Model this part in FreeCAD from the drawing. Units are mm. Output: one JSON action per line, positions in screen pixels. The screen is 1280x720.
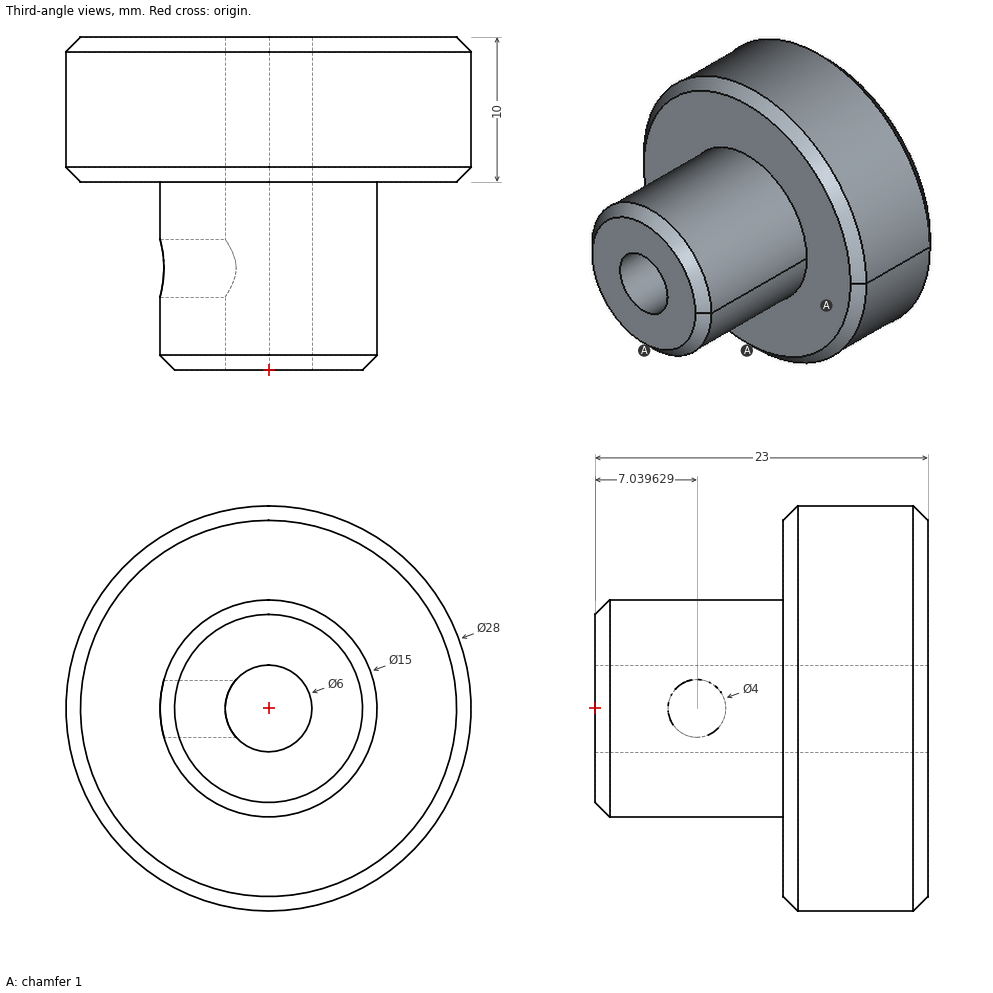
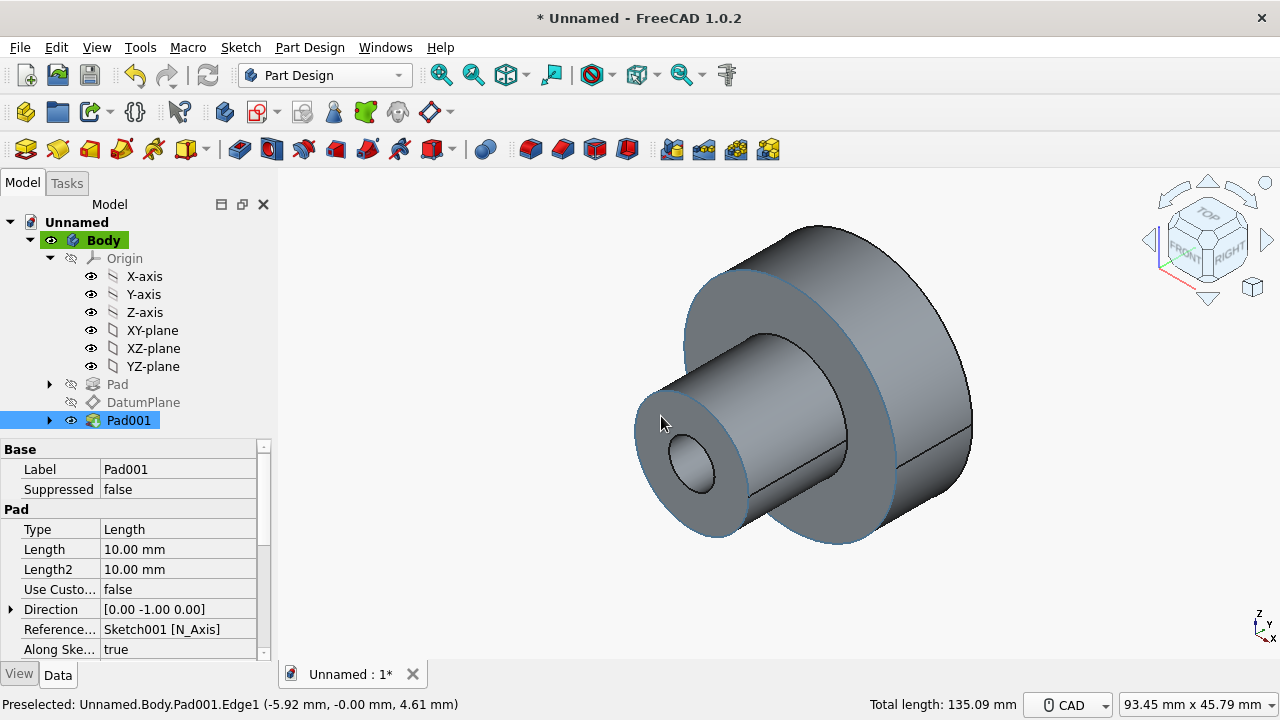
{"action": "key", "text": "2"}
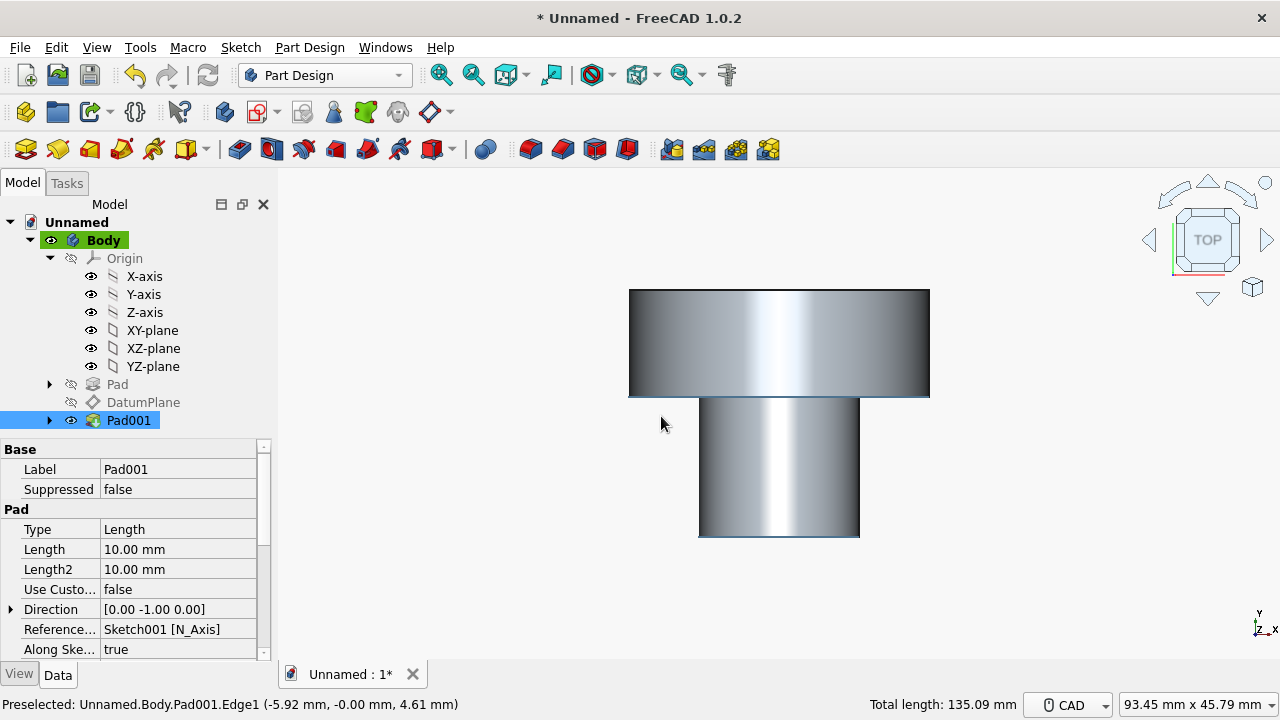
{"action": "left_click", "coordinate": [658, 289], "text": "ctrl"}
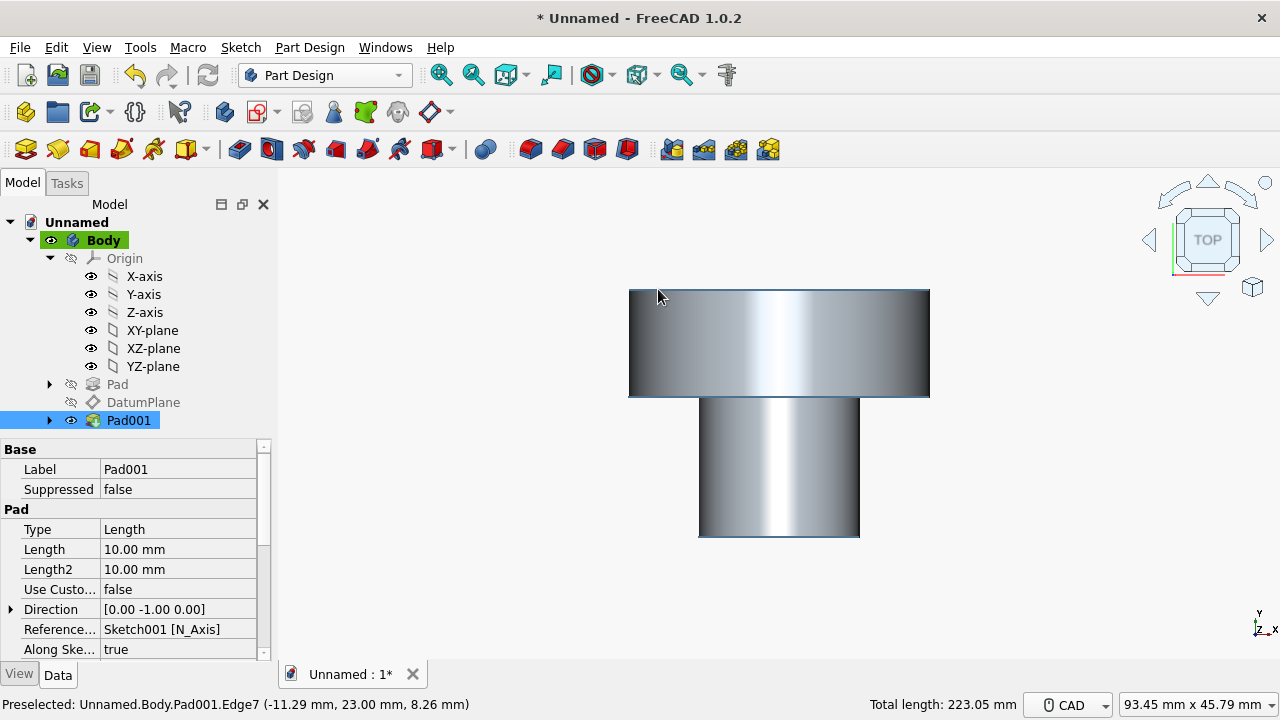
{"action": "left_click", "coordinate": [564, 150]}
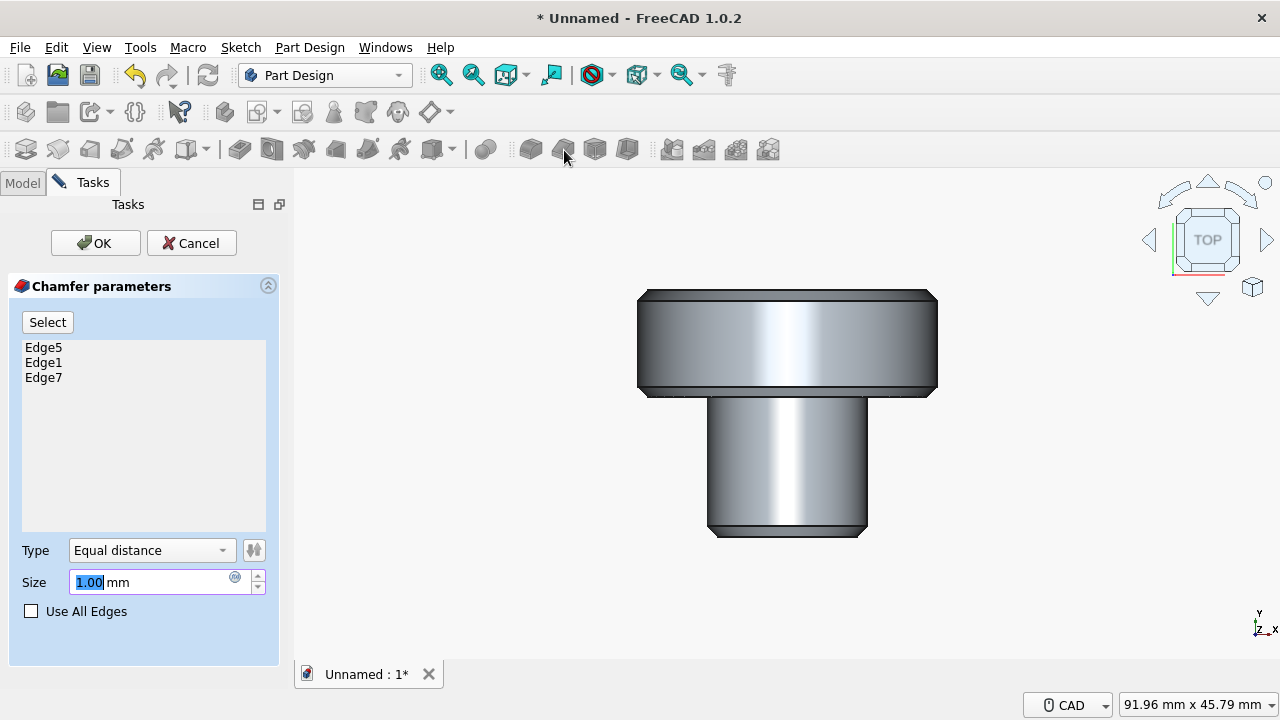
{"action": "type", "text": "1"}
{"action": "key", "text": "Tab"}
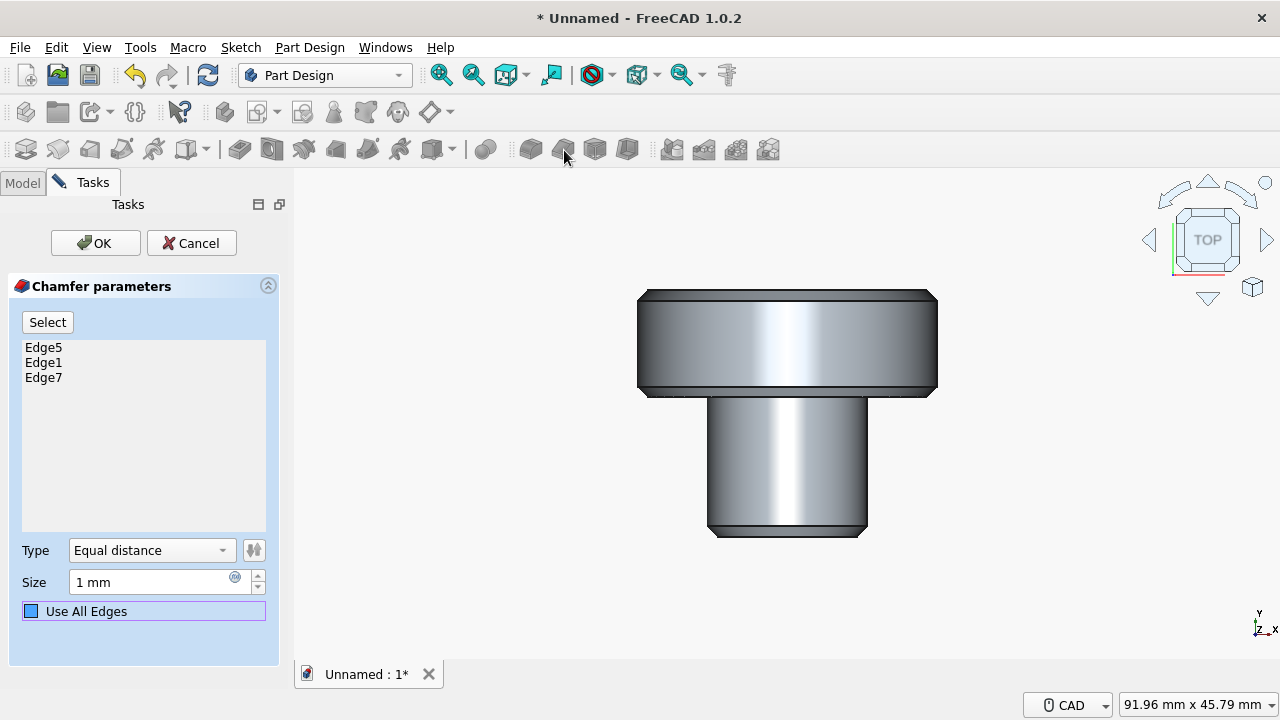
{"action": "left_click", "coordinate": [96, 243]}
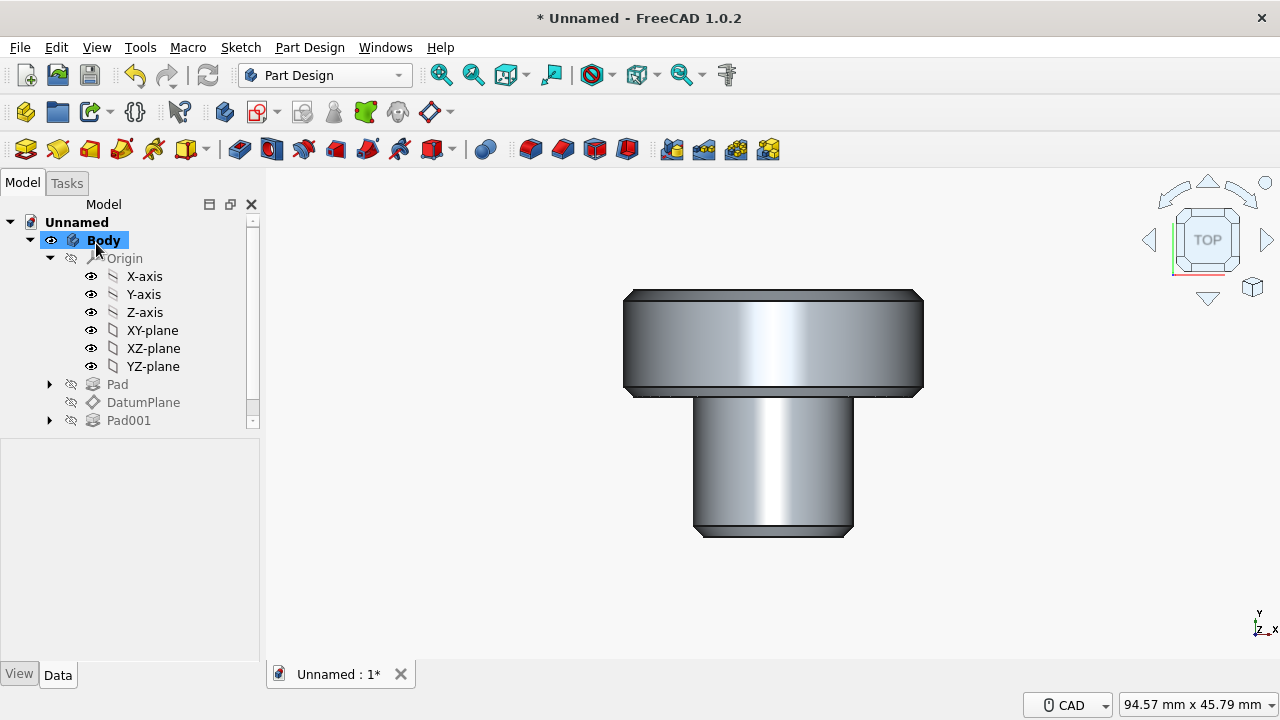
{"action": "left_click", "coordinate": [258, 112]}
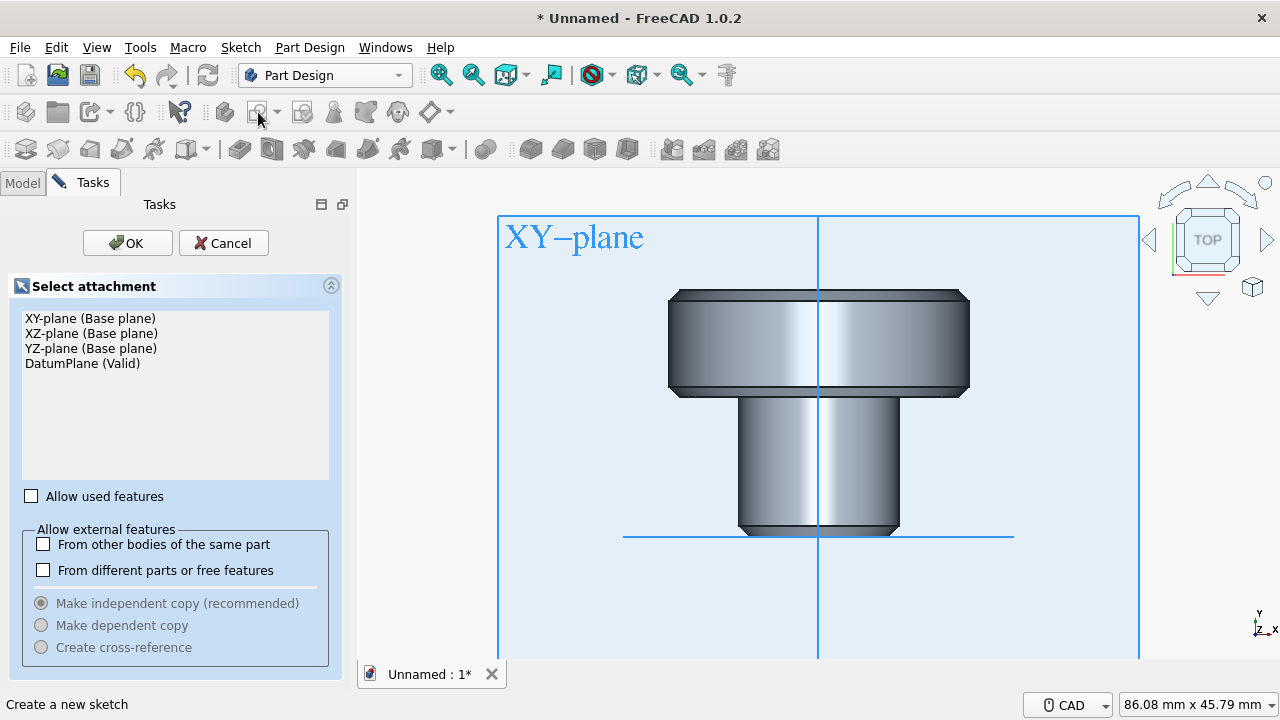
{"action": "left_click", "coordinate": [82, 348]}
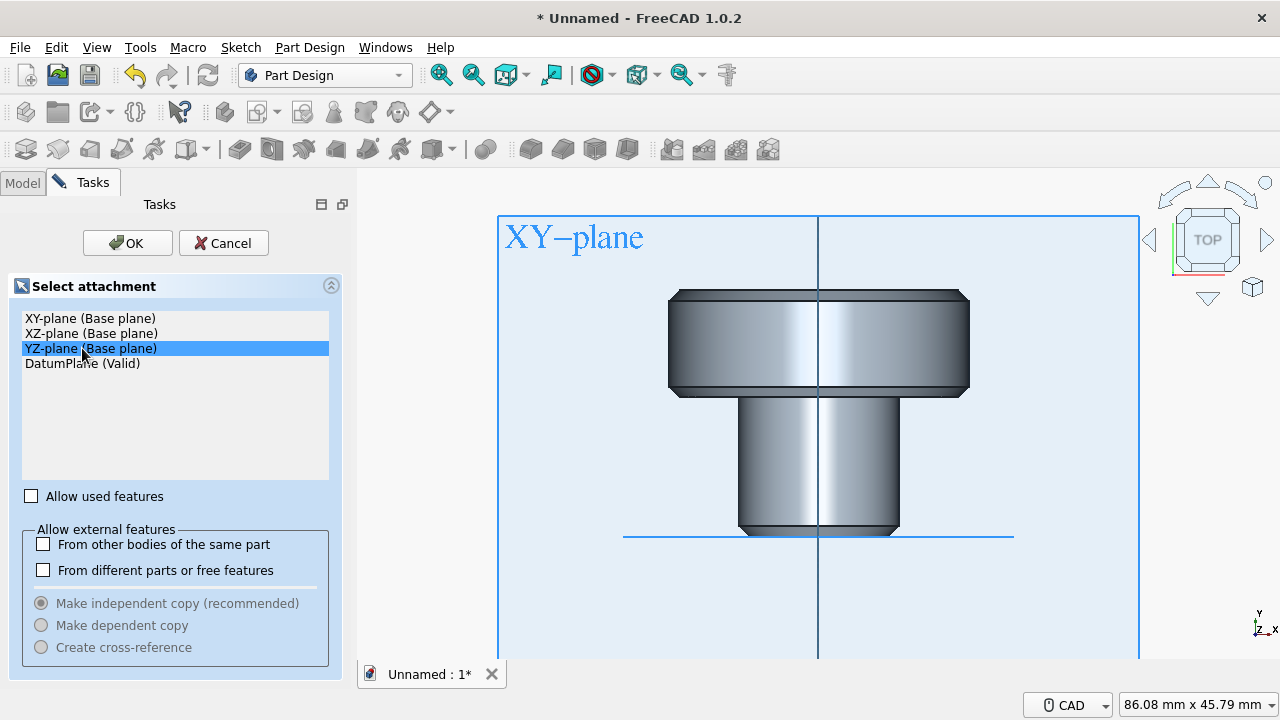
{"action": "left_click", "coordinate": [128, 243]}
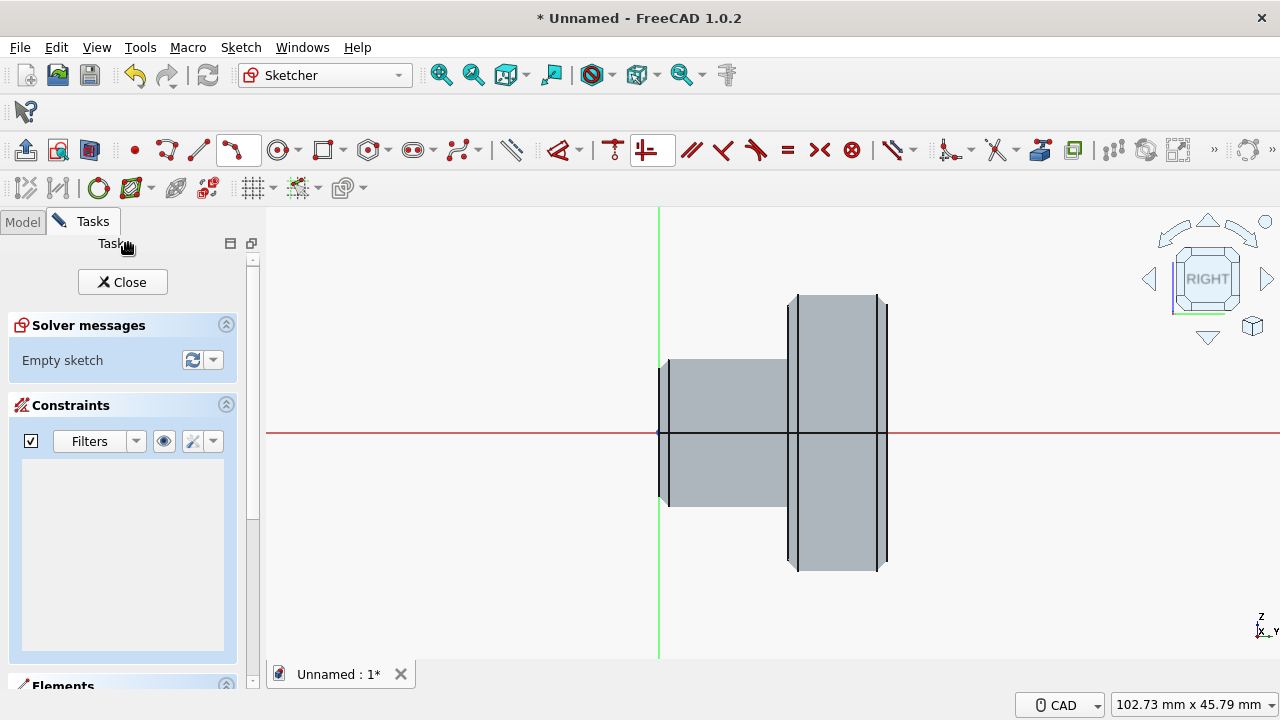
{"action": "left_click", "coordinate": [90, 150]}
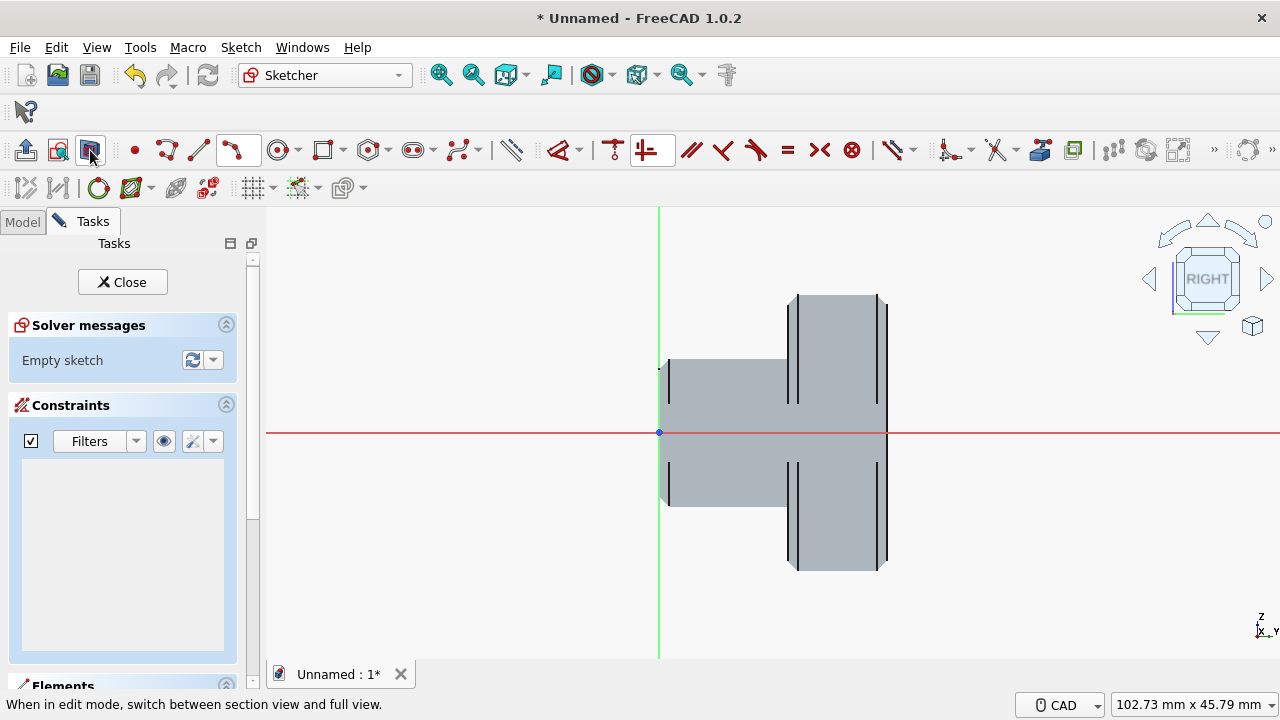
{"action": "scroll", "coordinate": [704, 433], "scroll_direction": "up", "scroll_amount": 9}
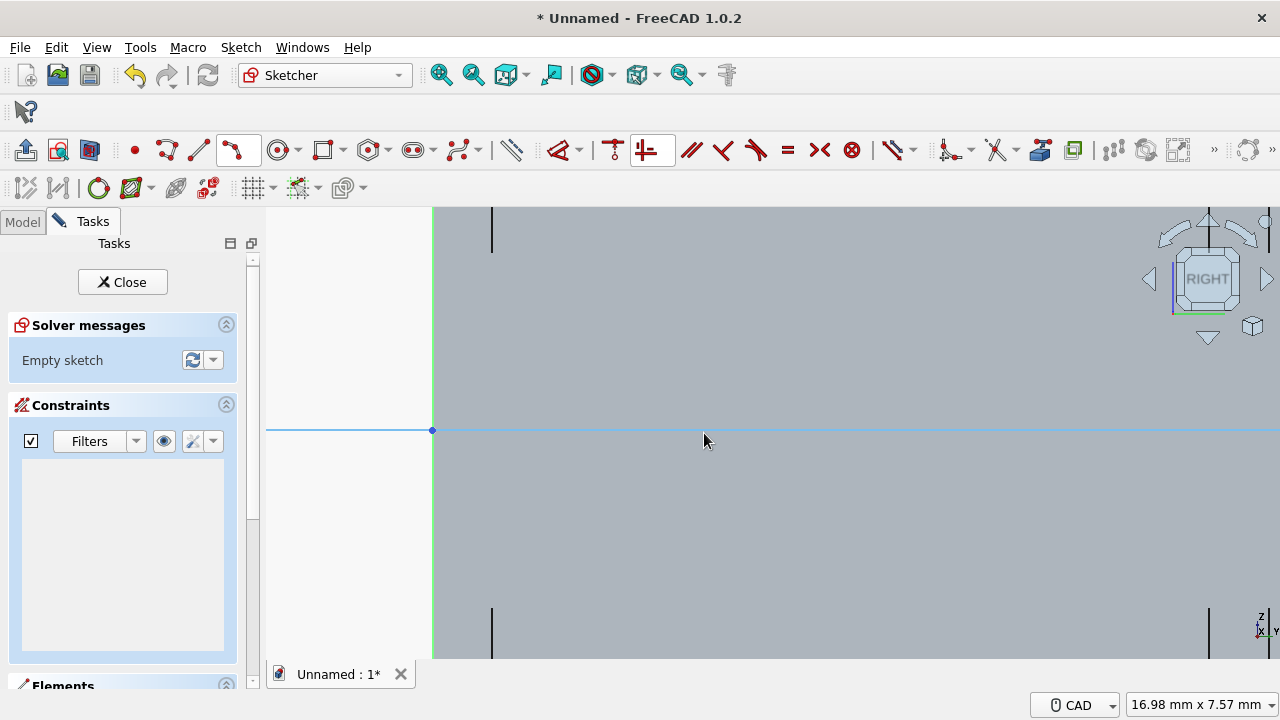
{"action": "left_click", "coordinate": [278, 150]}